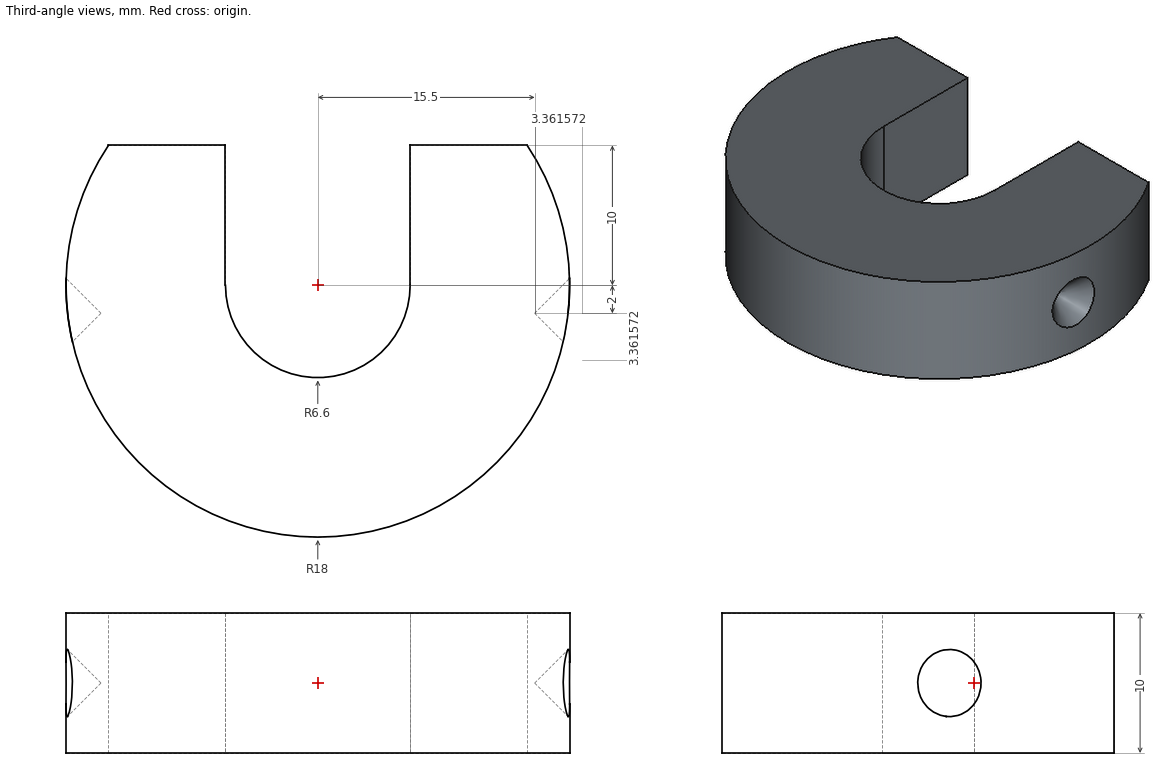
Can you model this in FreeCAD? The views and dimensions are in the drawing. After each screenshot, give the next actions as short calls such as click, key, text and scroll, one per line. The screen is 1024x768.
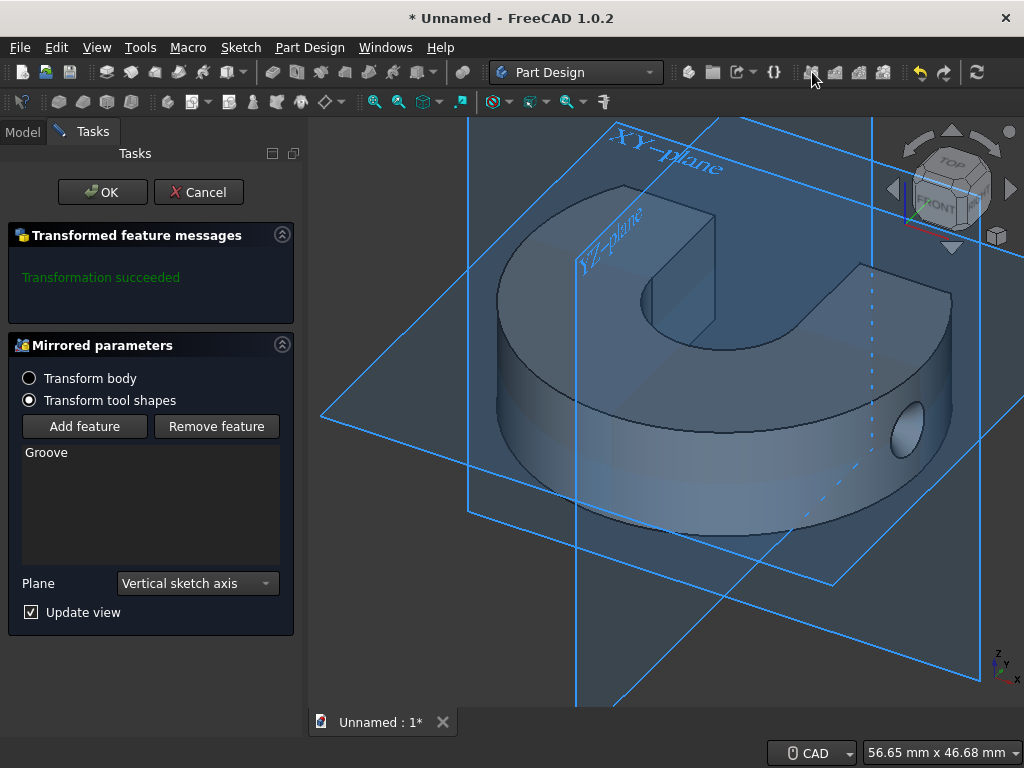
click(198, 584)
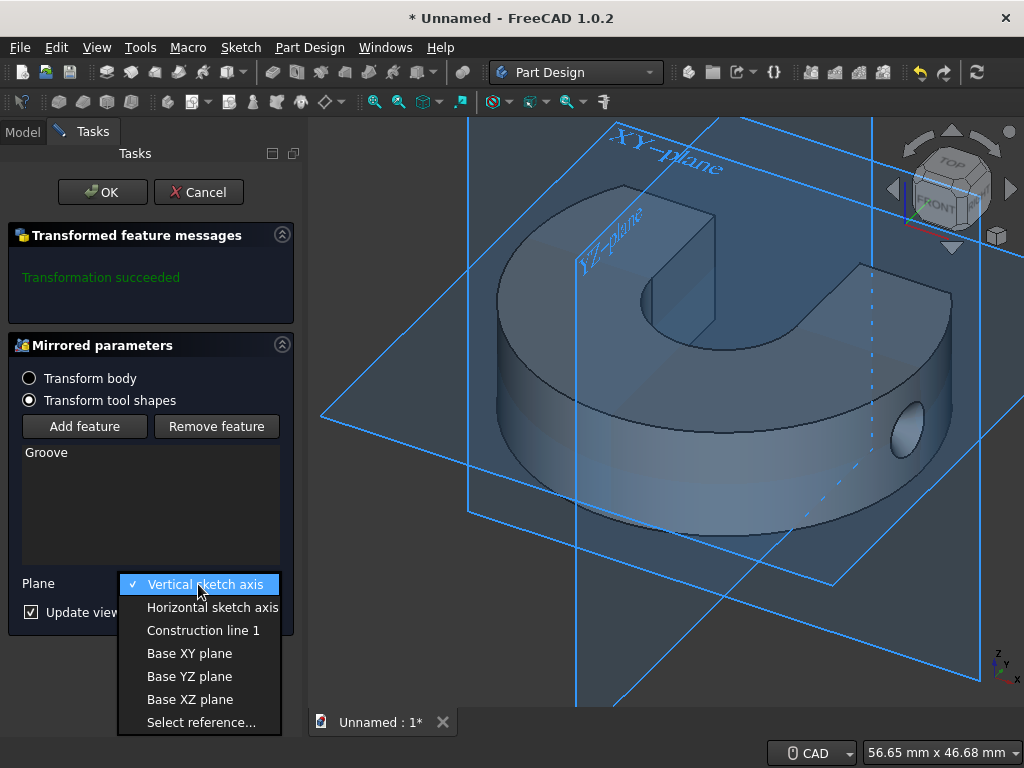
click(198, 676)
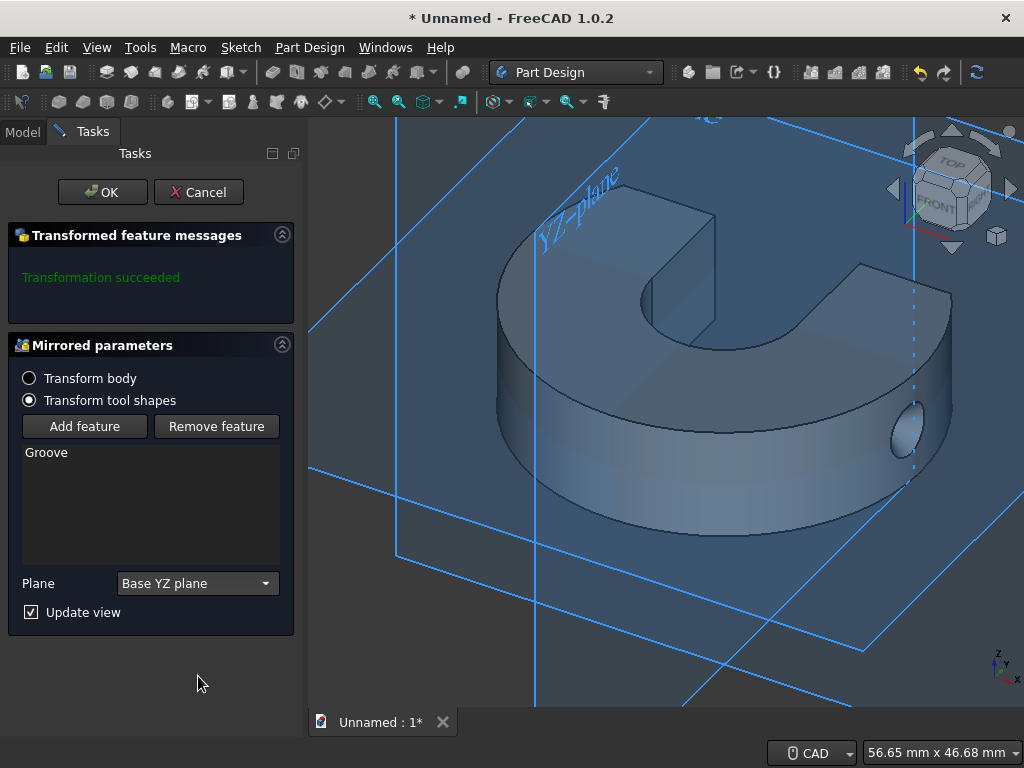
click(103, 192)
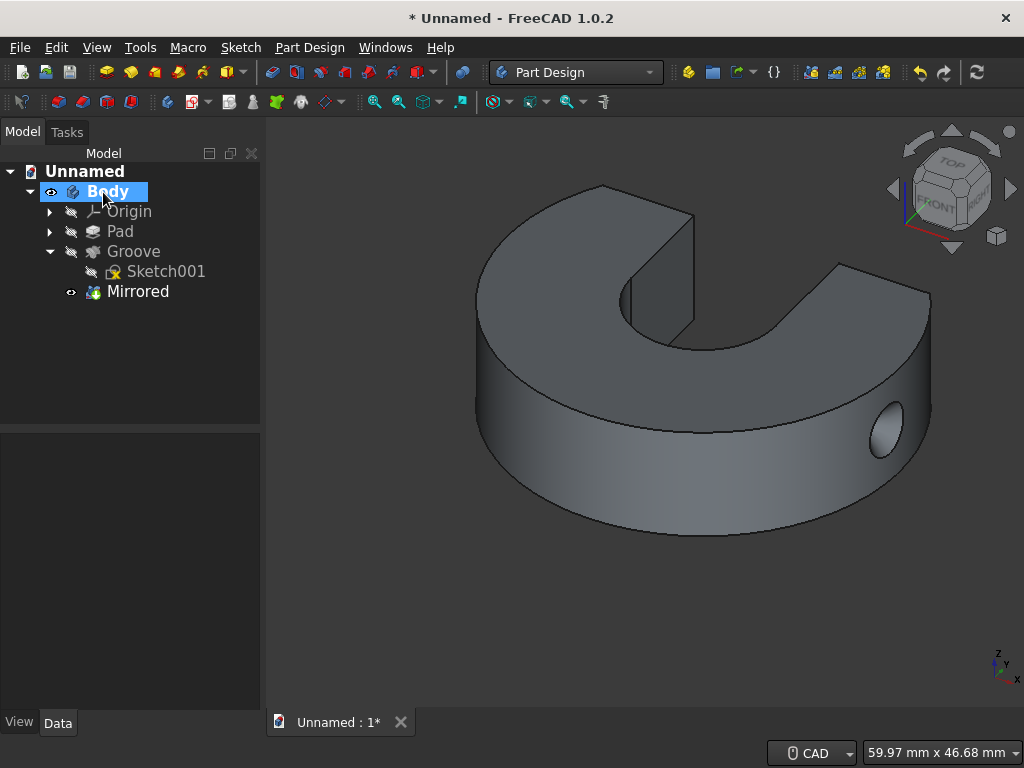
key(0)